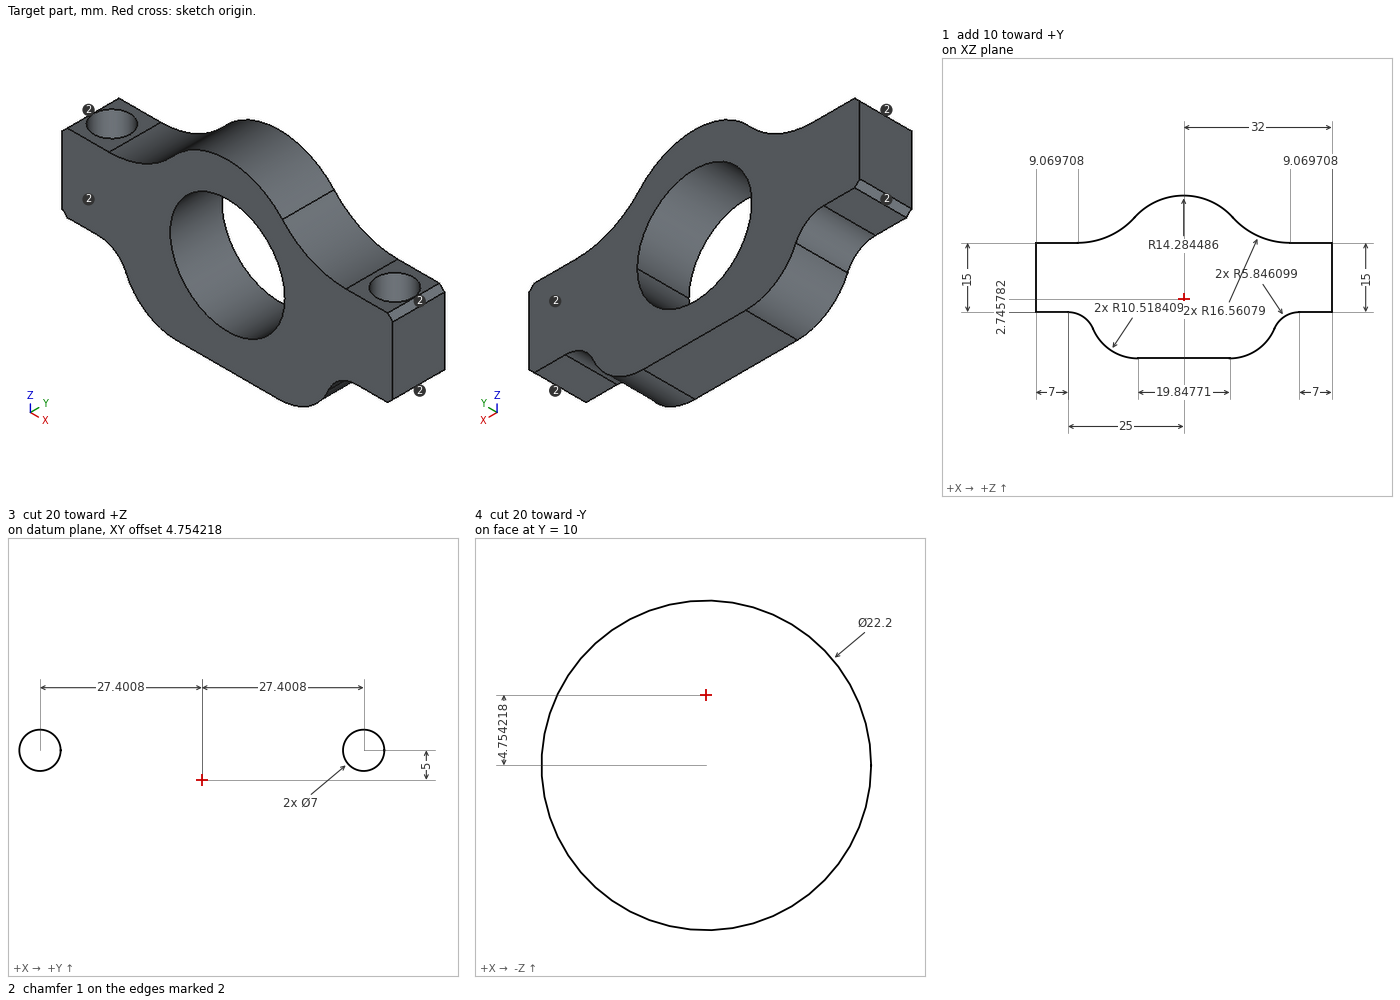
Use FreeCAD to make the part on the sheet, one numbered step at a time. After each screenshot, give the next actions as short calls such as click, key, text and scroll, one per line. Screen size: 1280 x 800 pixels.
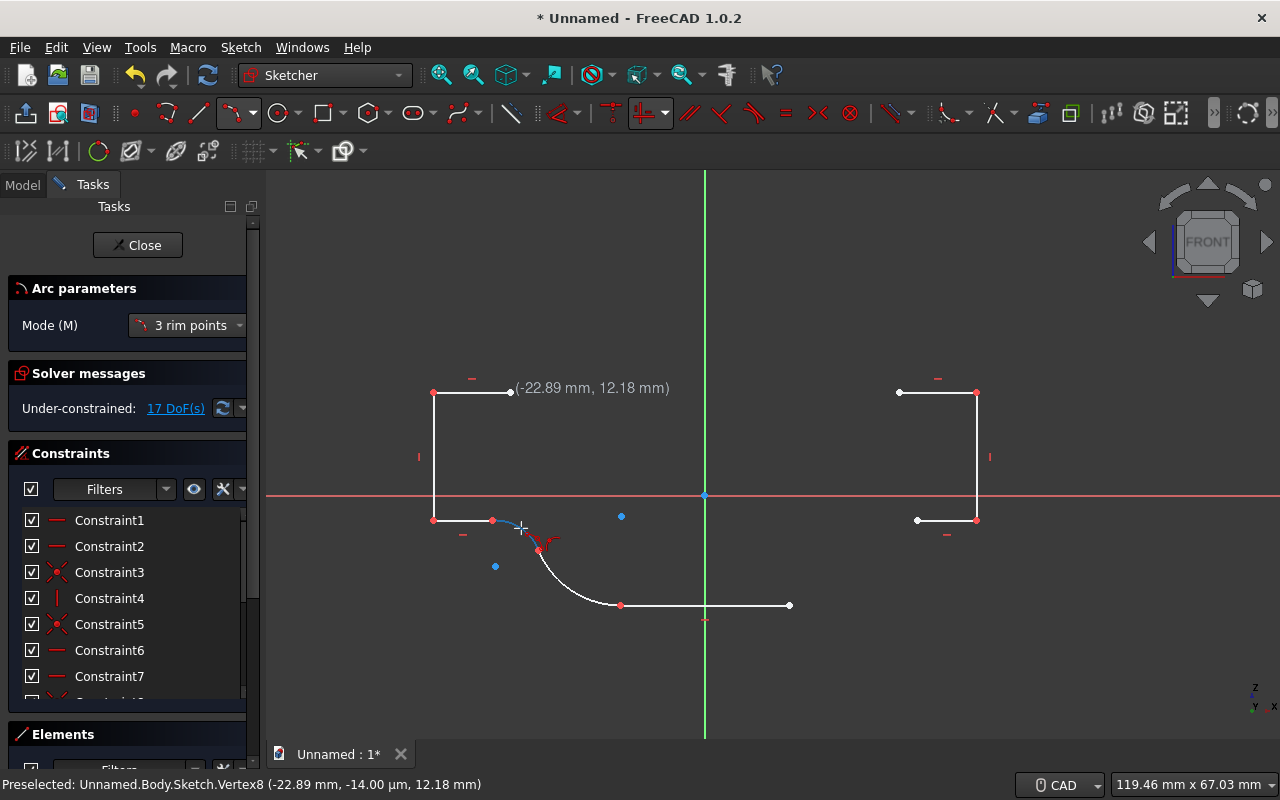
click(615, 345)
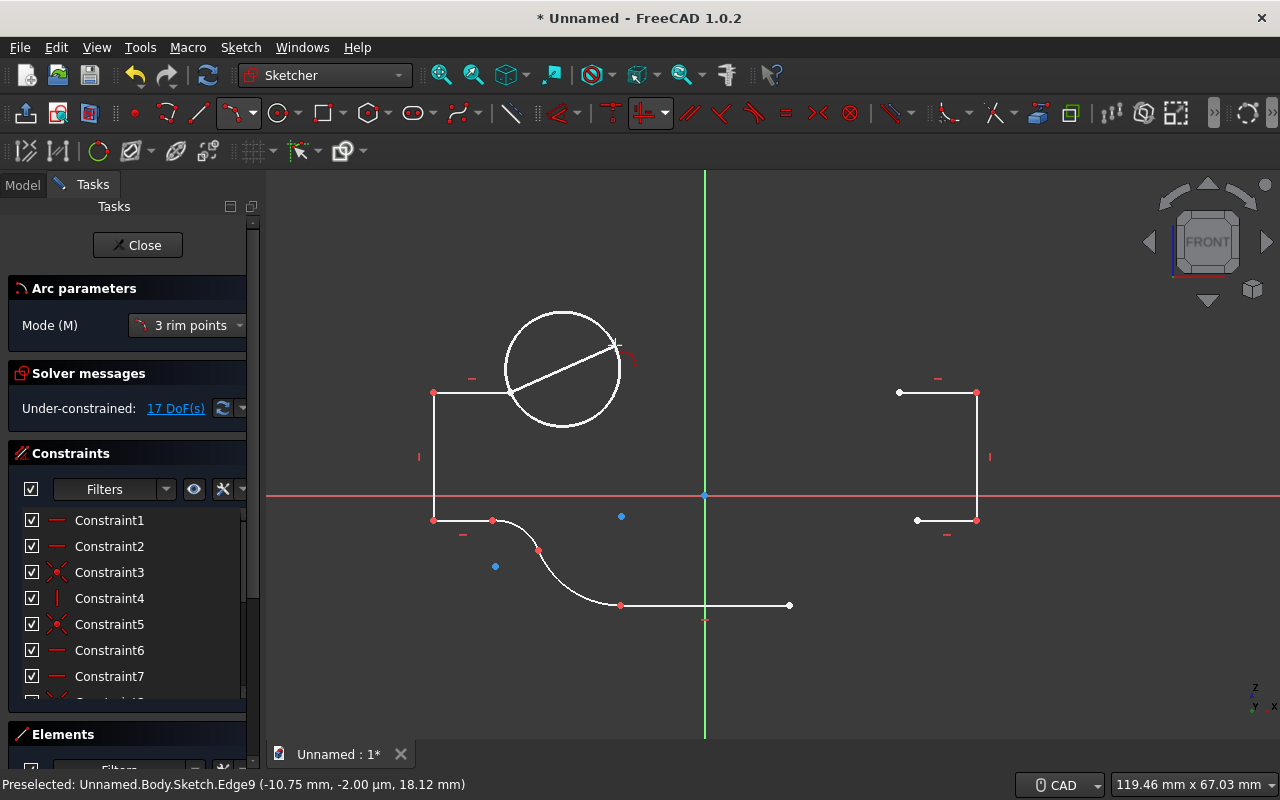
scroll(567, 380, up, 2)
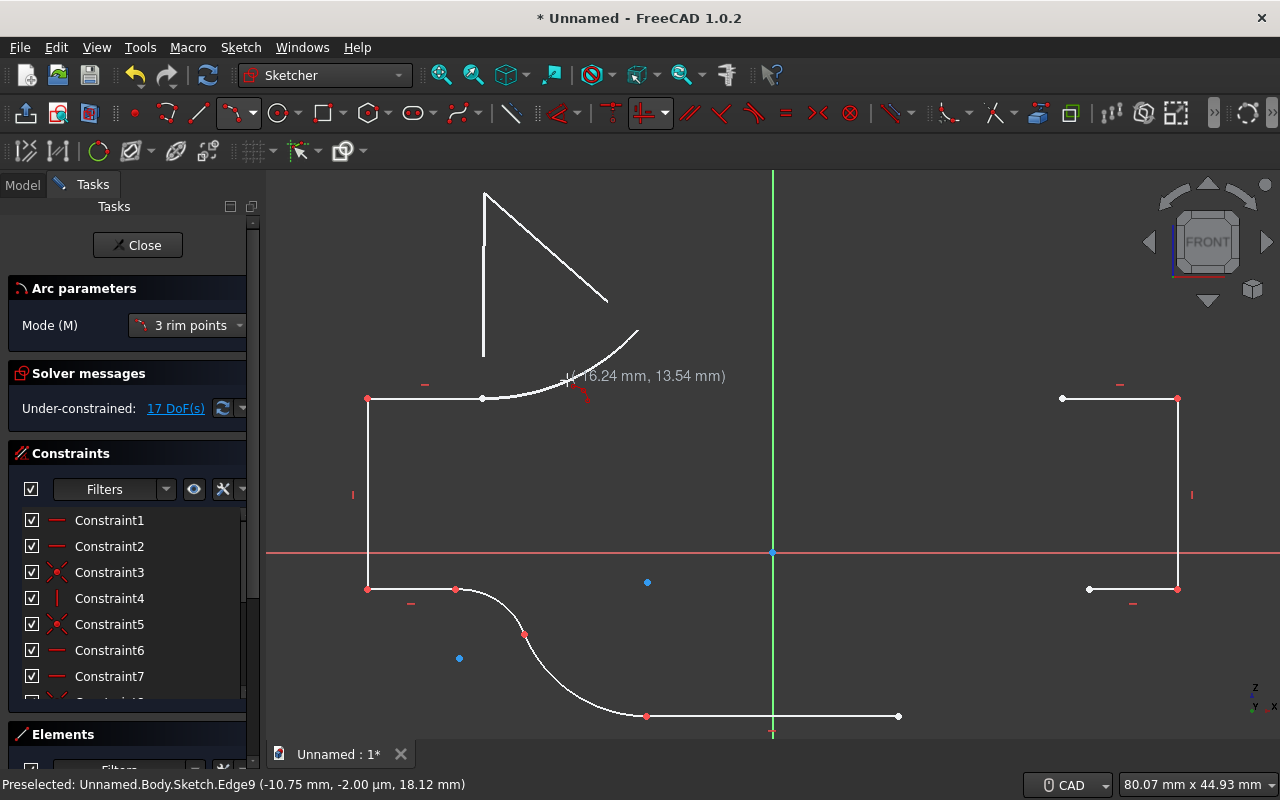
click(567, 379)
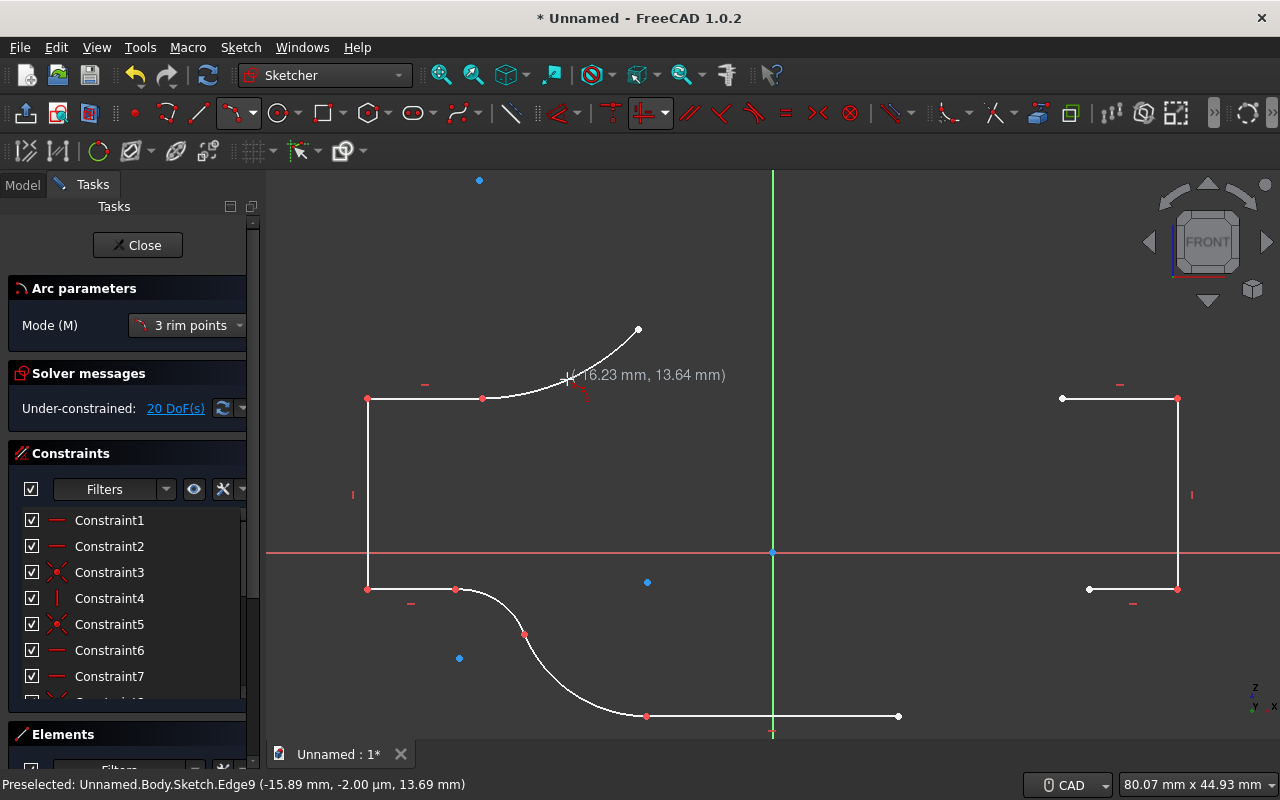
click(638, 329)
click(907, 328)
click(803, 271)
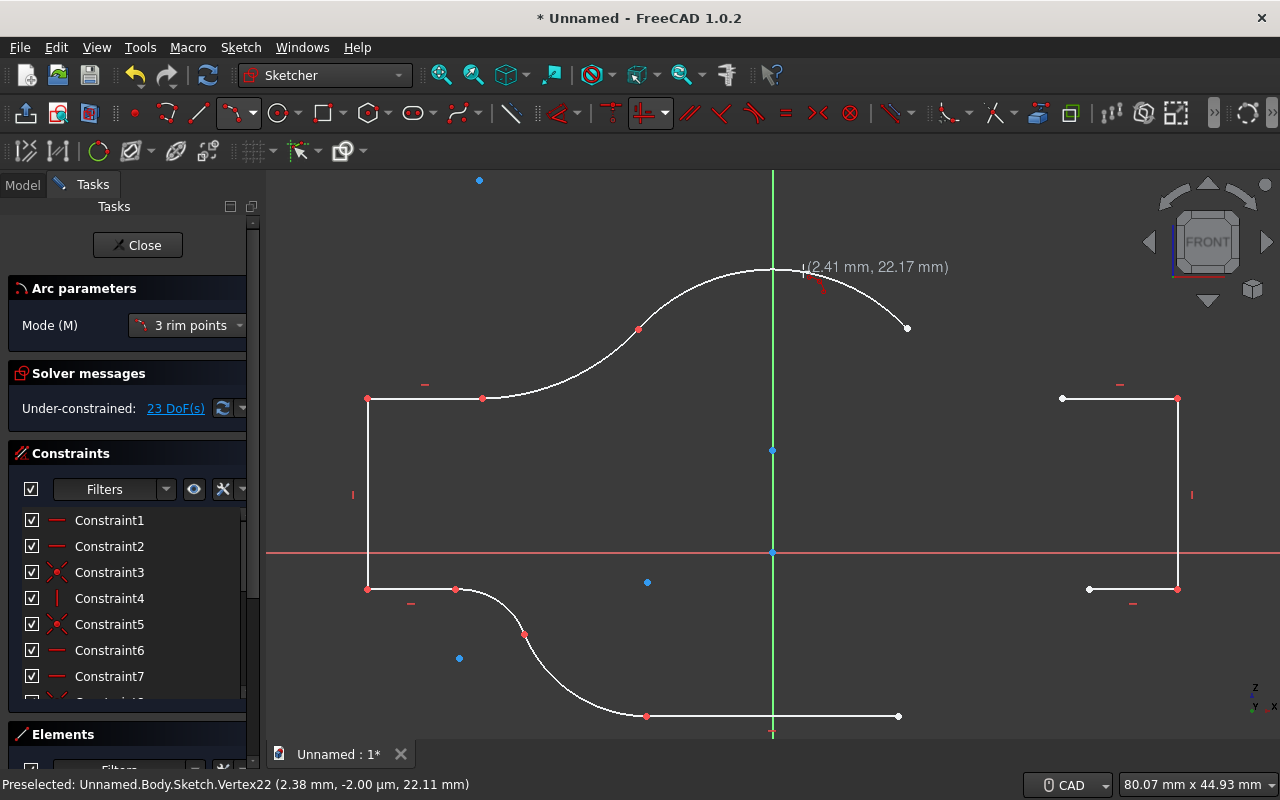
click(907, 329)
click(1063, 399)
click(978, 379)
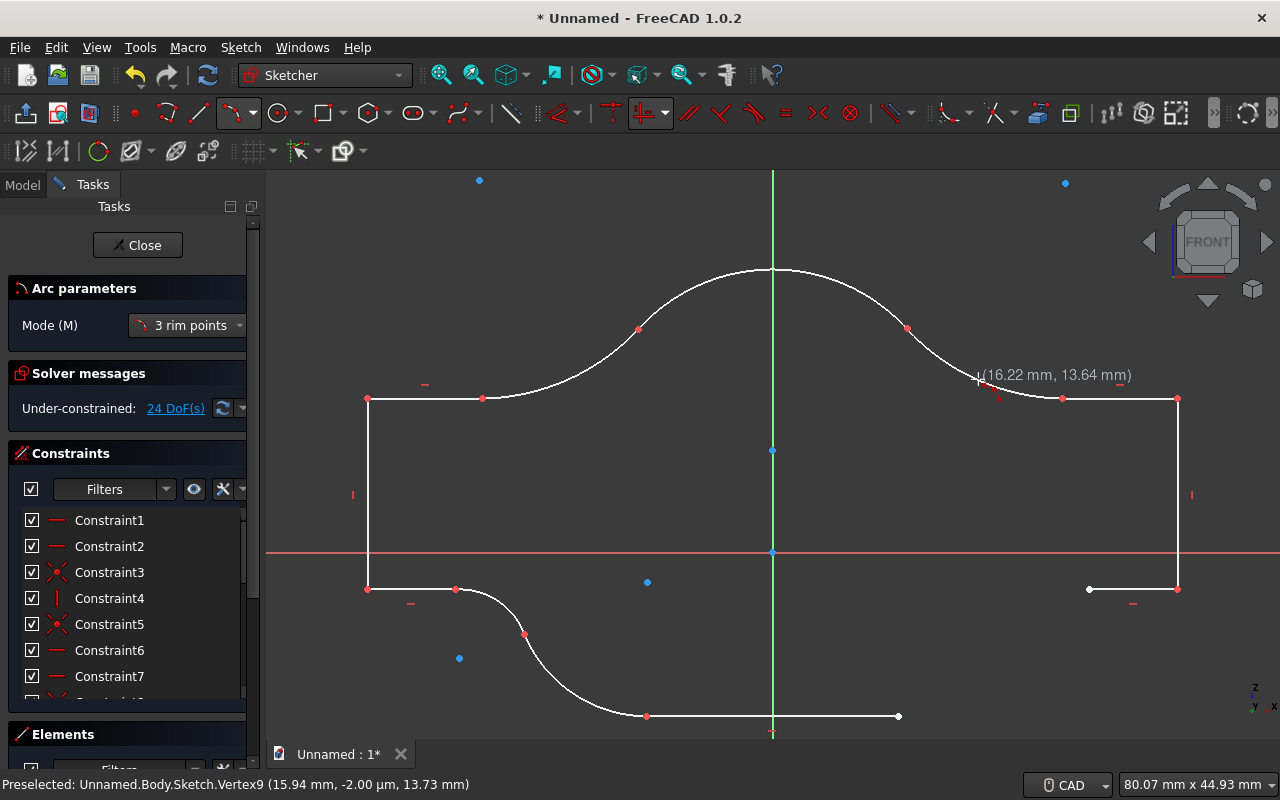
click(1090, 589)
click(1021, 633)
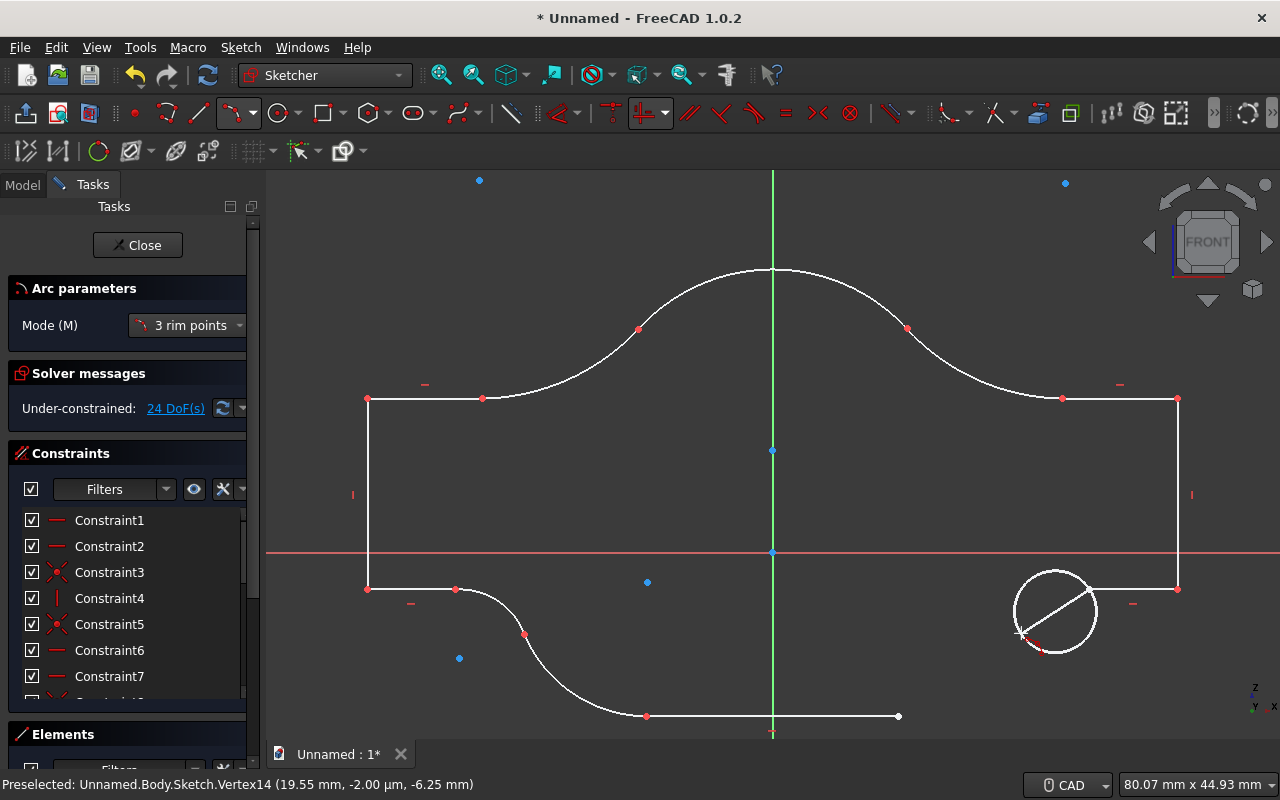
scroll(1048, 600, up, 2)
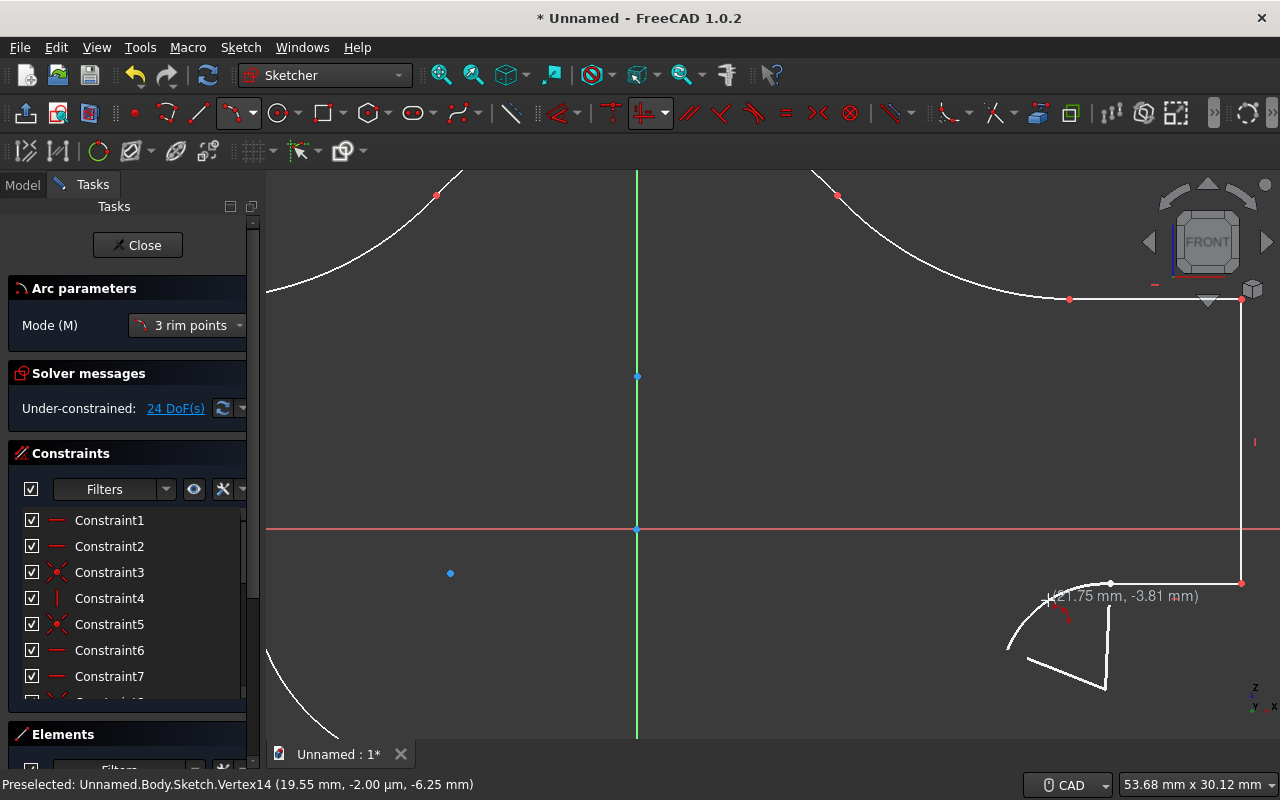
click(1048, 599)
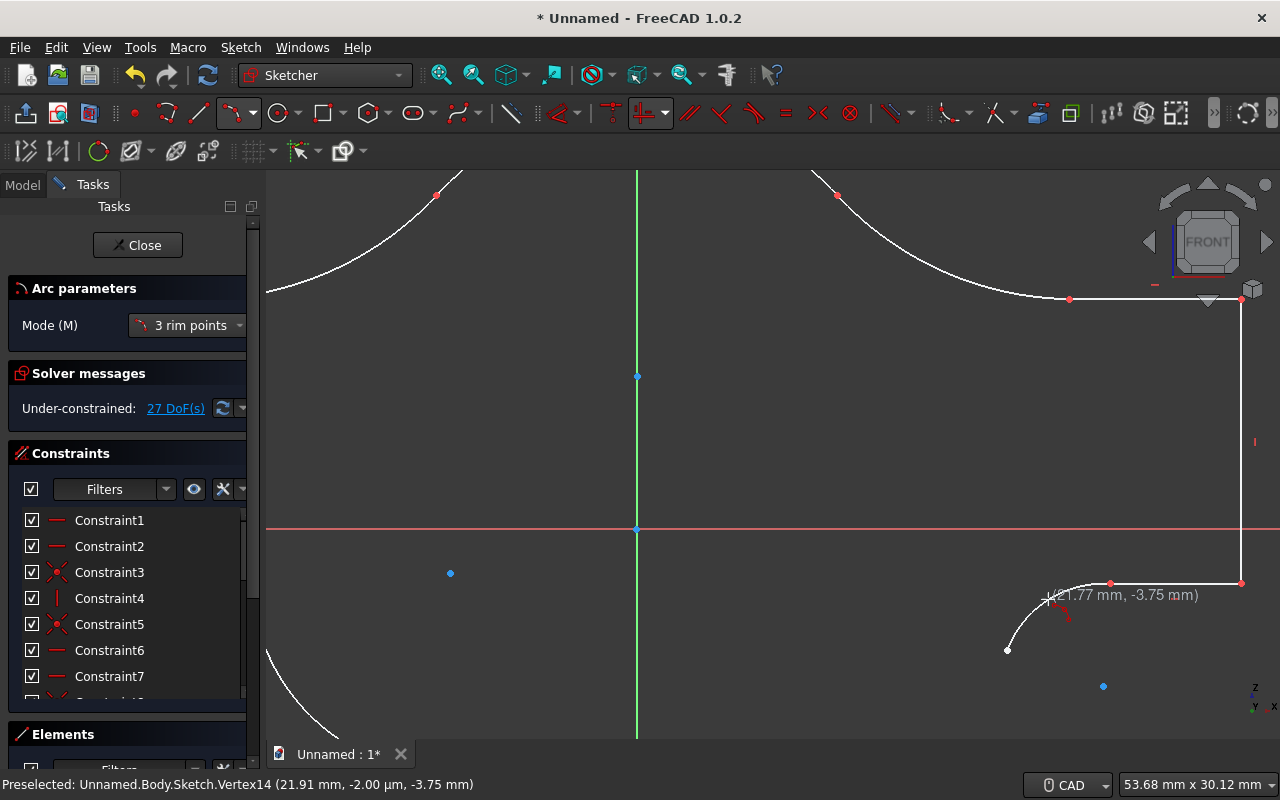
click(1007, 650)